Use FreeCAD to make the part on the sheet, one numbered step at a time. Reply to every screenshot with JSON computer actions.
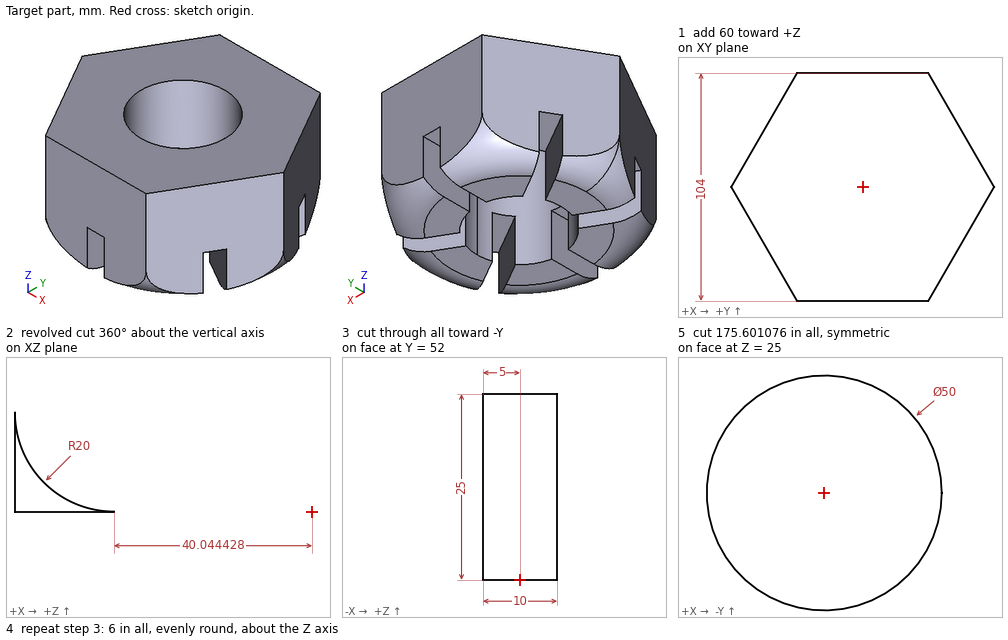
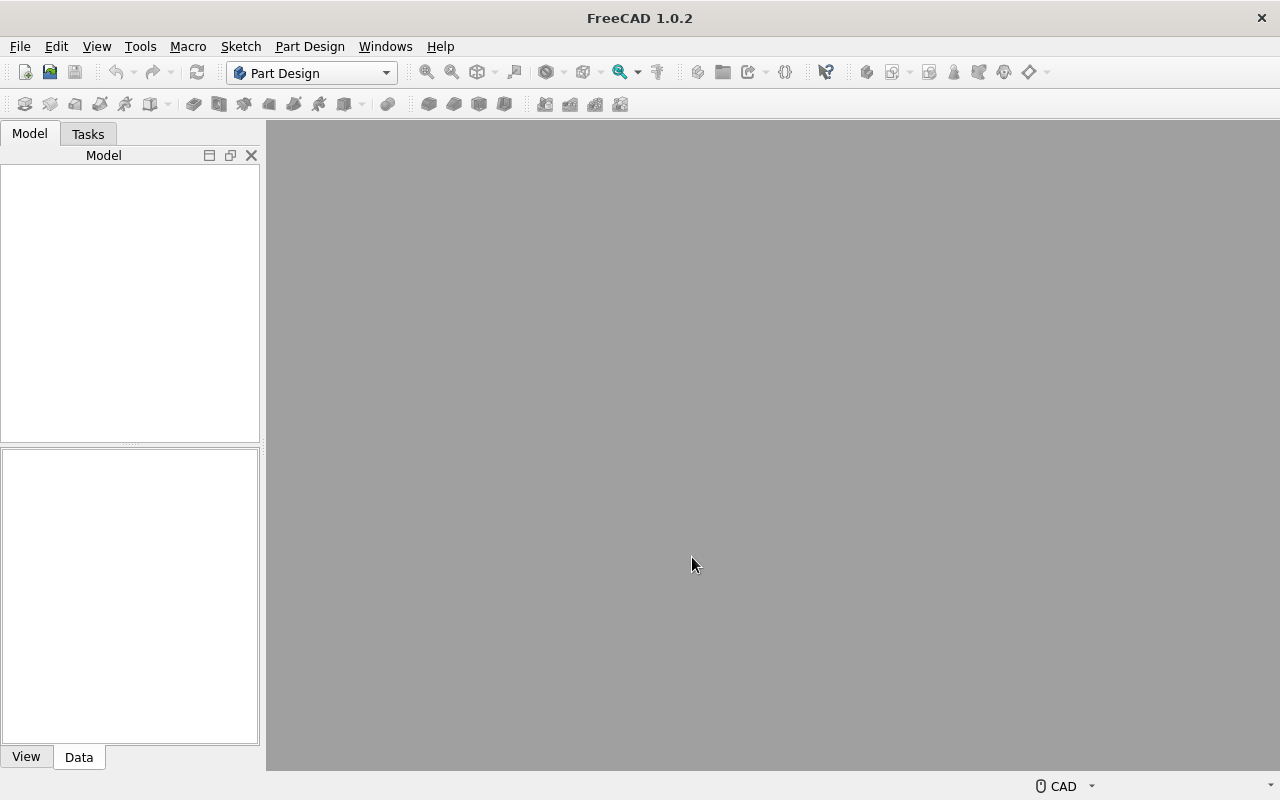
{"action": "left_click", "coordinate": [25, 72]}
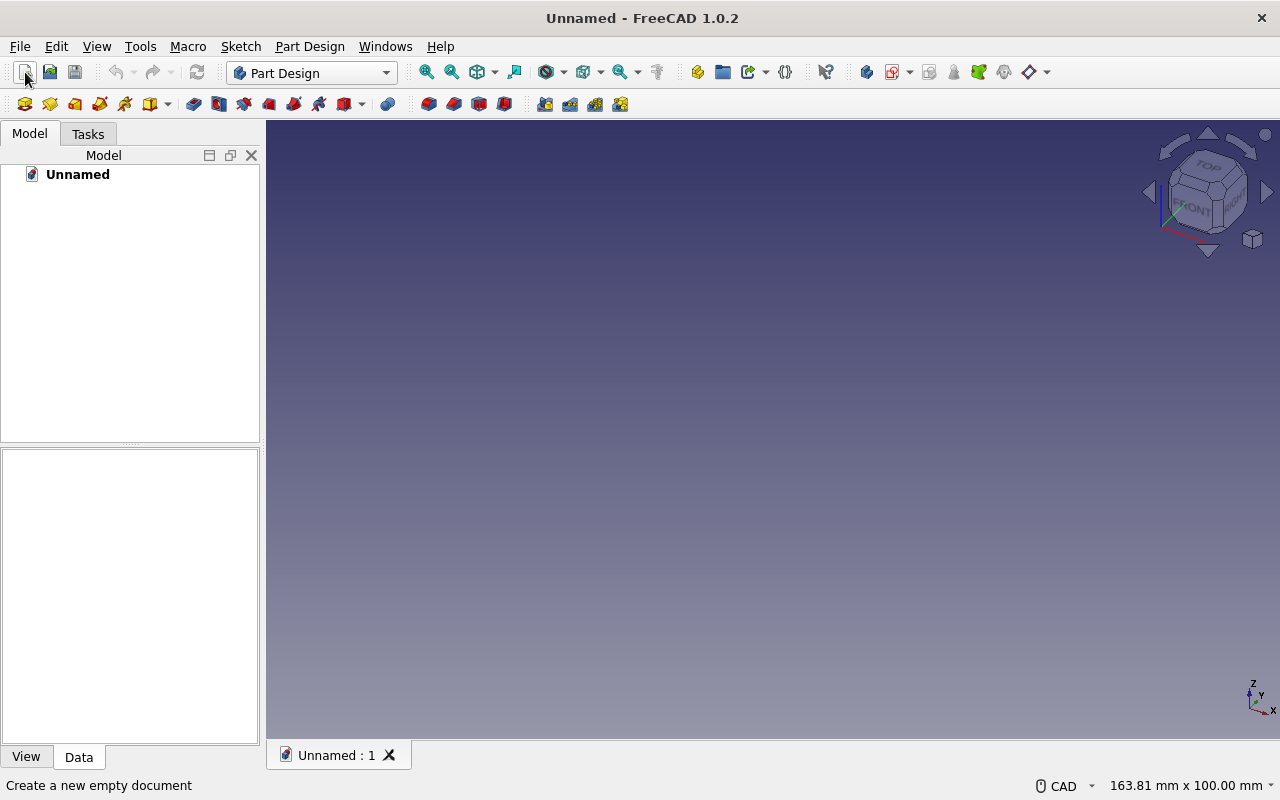
{"action": "left_click", "coordinate": [892, 72]}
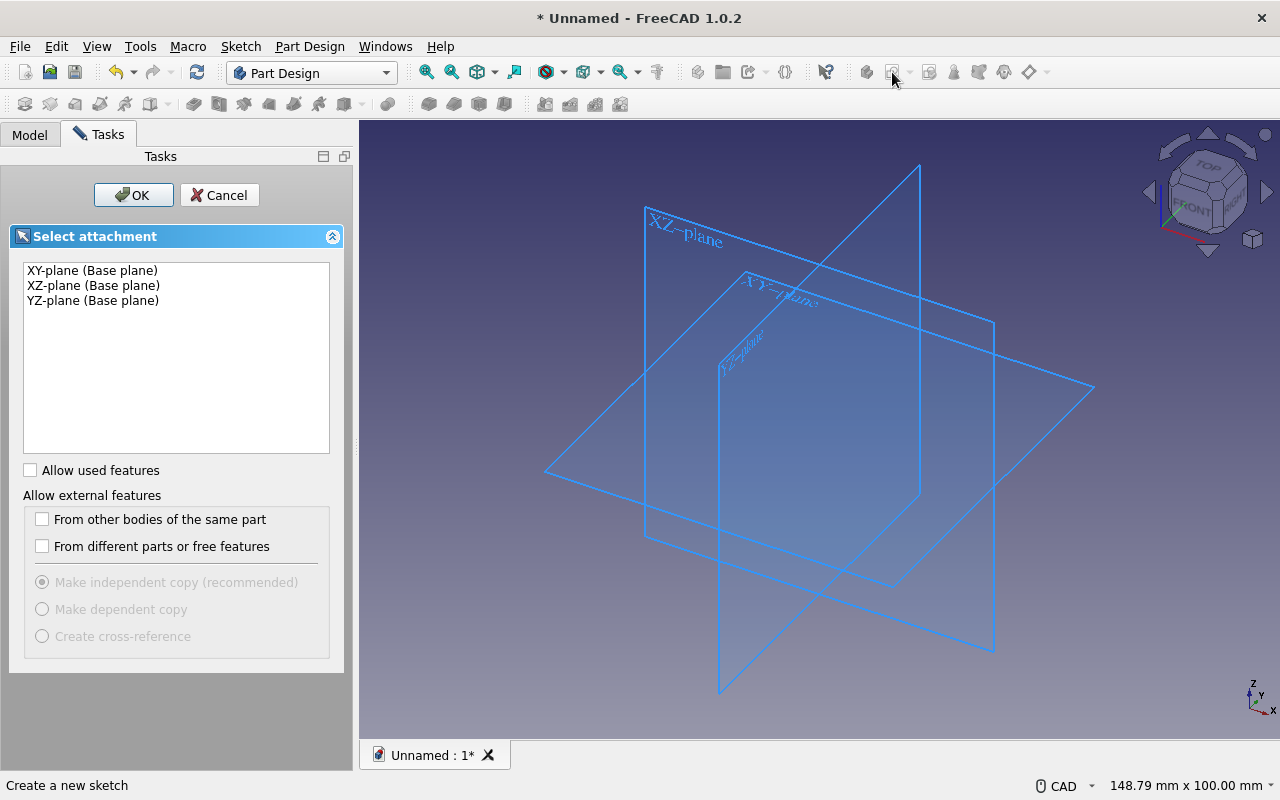
{"action": "left_click", "coordinate": [84, 270]}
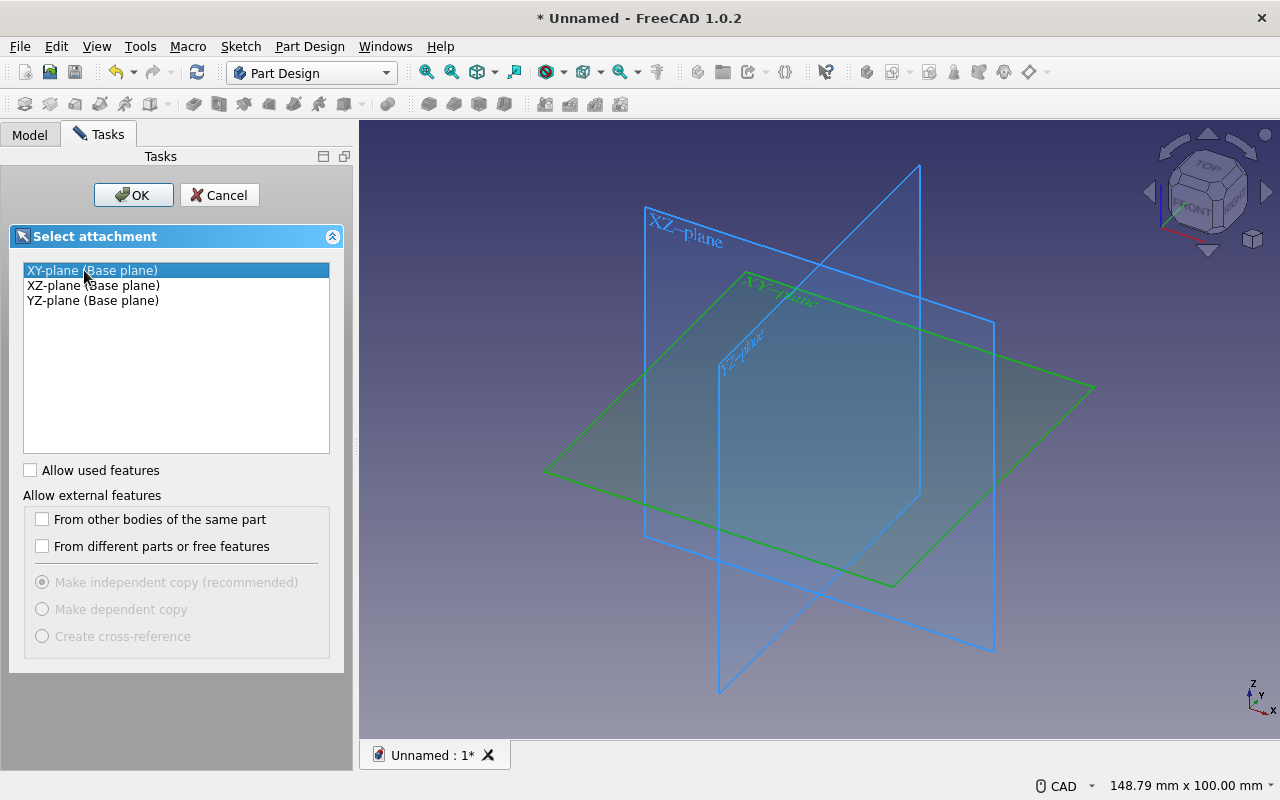
{"action": "left_click", "coordinate": [134, 195]}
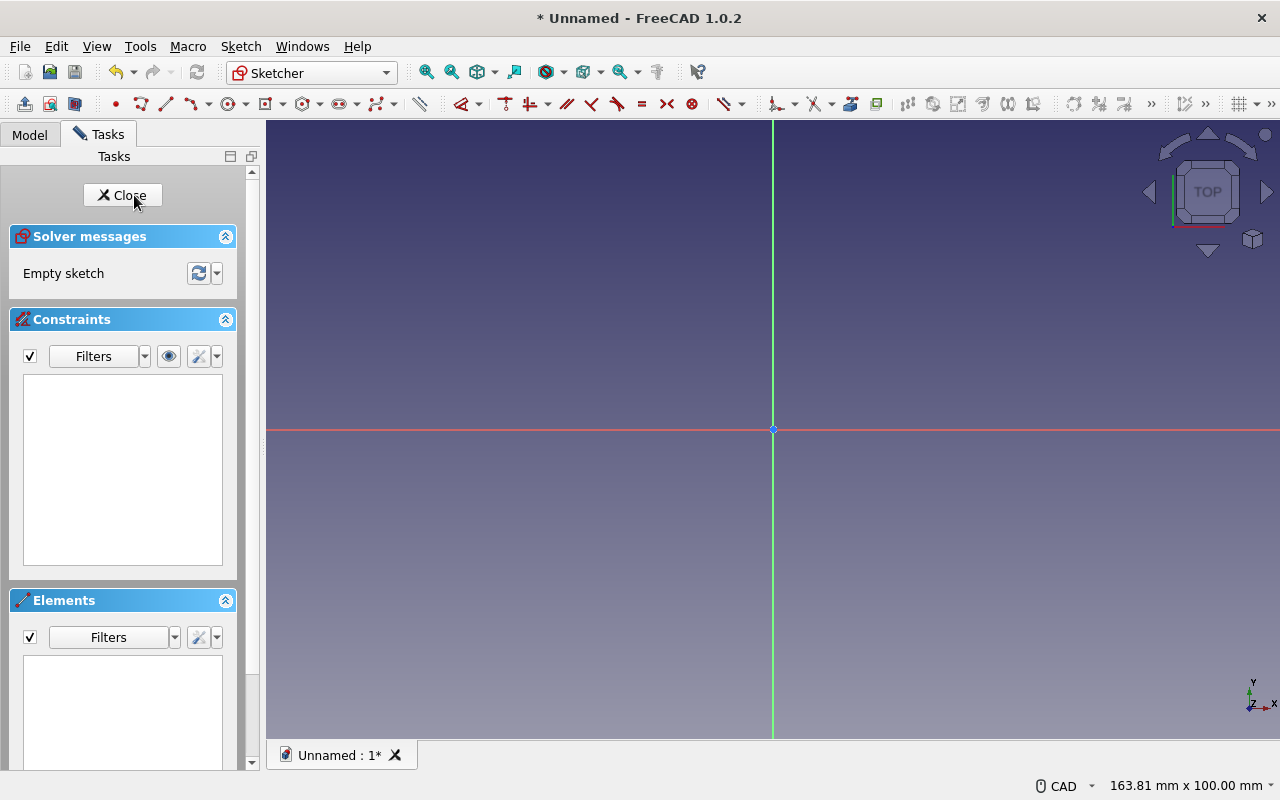
{"action": "scroll", "coordinate": [565, 429], "scroll_direction": "down", "scroll_amount": 2}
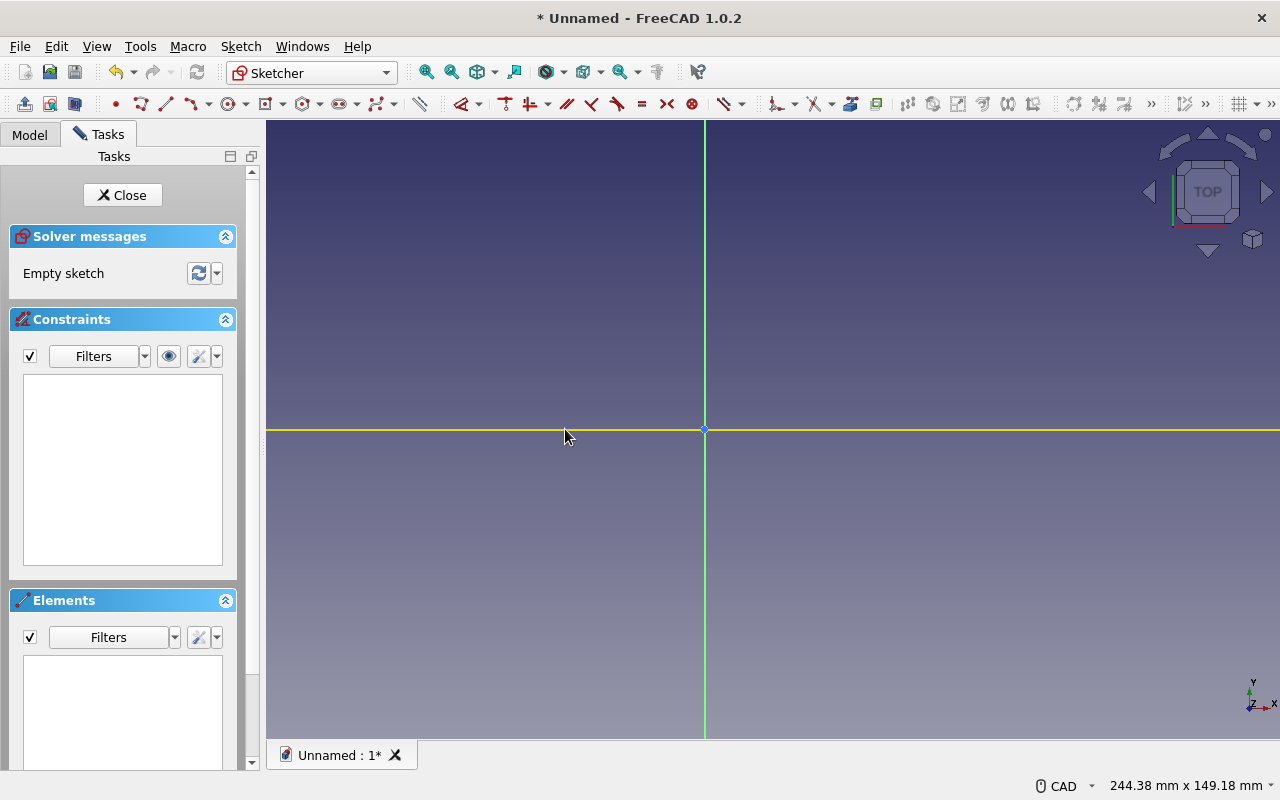
{"action": "left_click", "coordinate": [302, 104]}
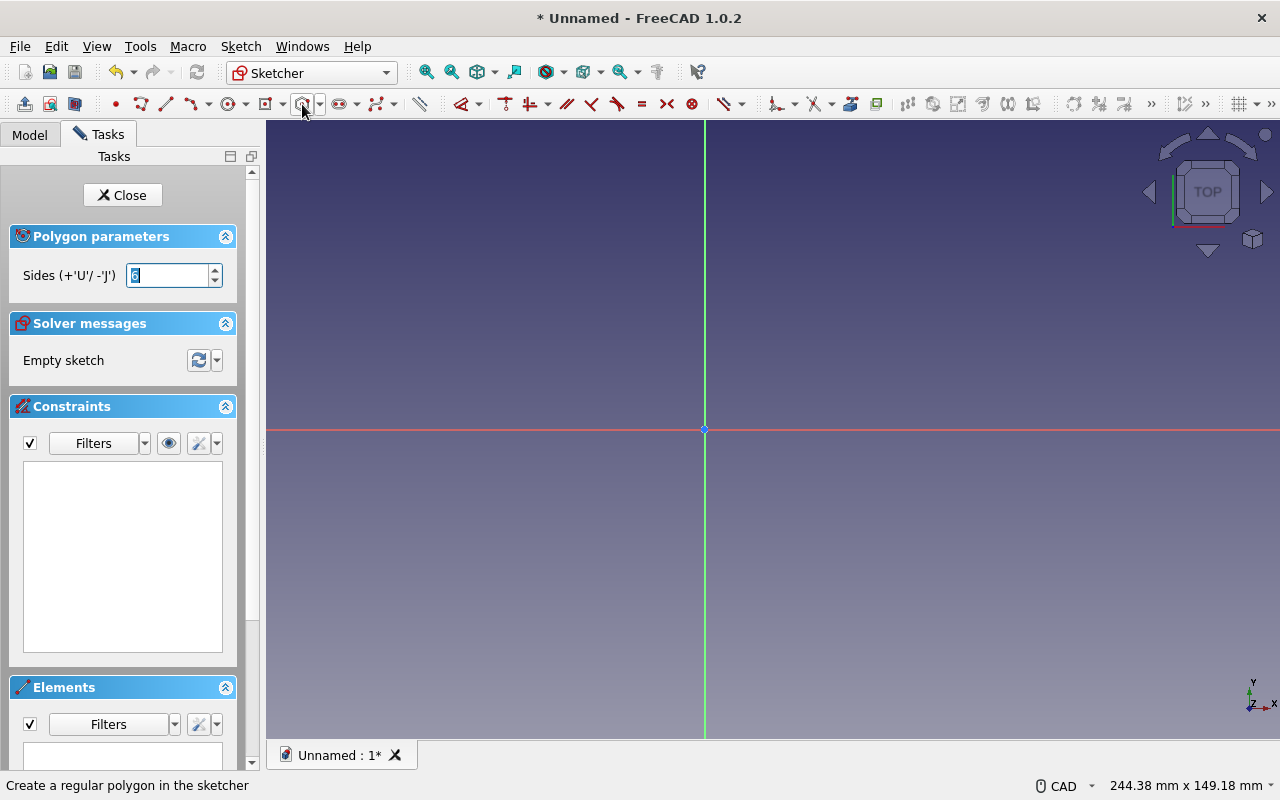
{"action": "left_click", "coordinate": [705, 430]}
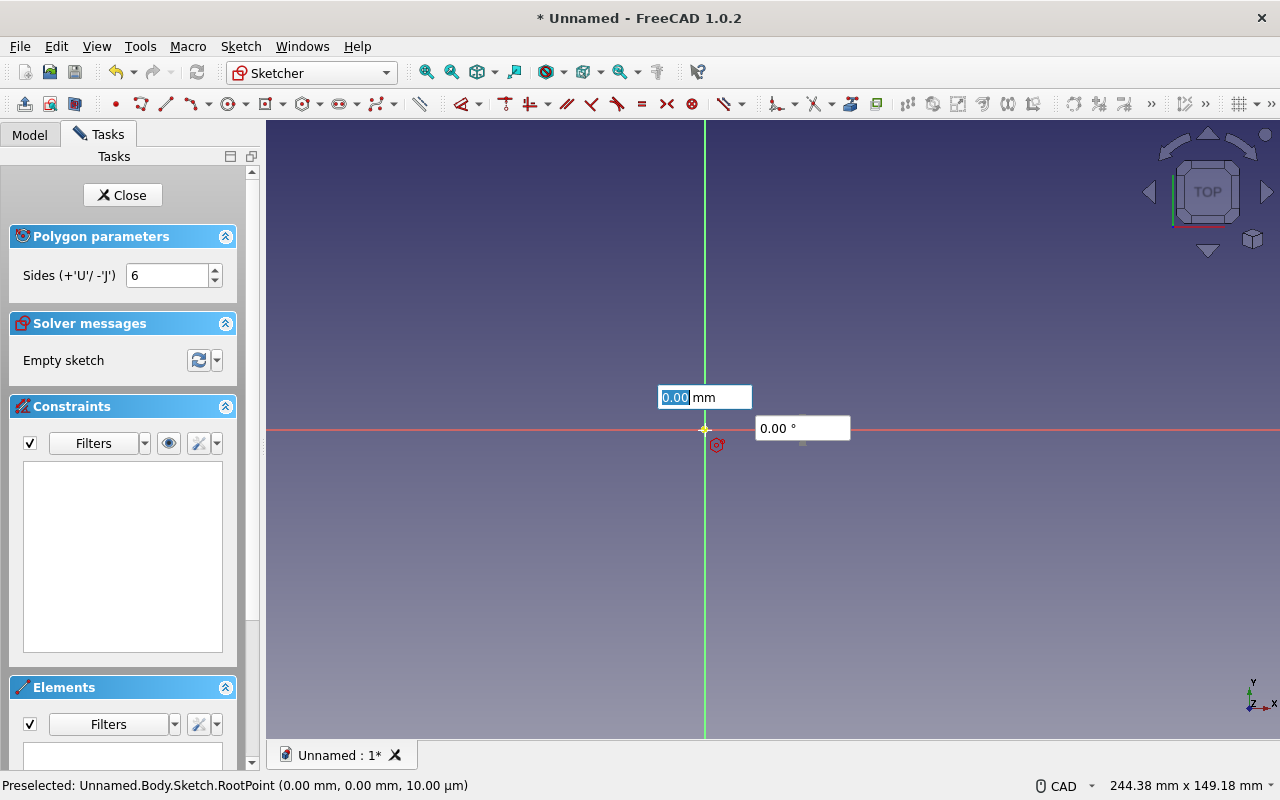
{"action": "left_click", "coordinate": [954, 430]}
{"action": "key", "text": "Escape"}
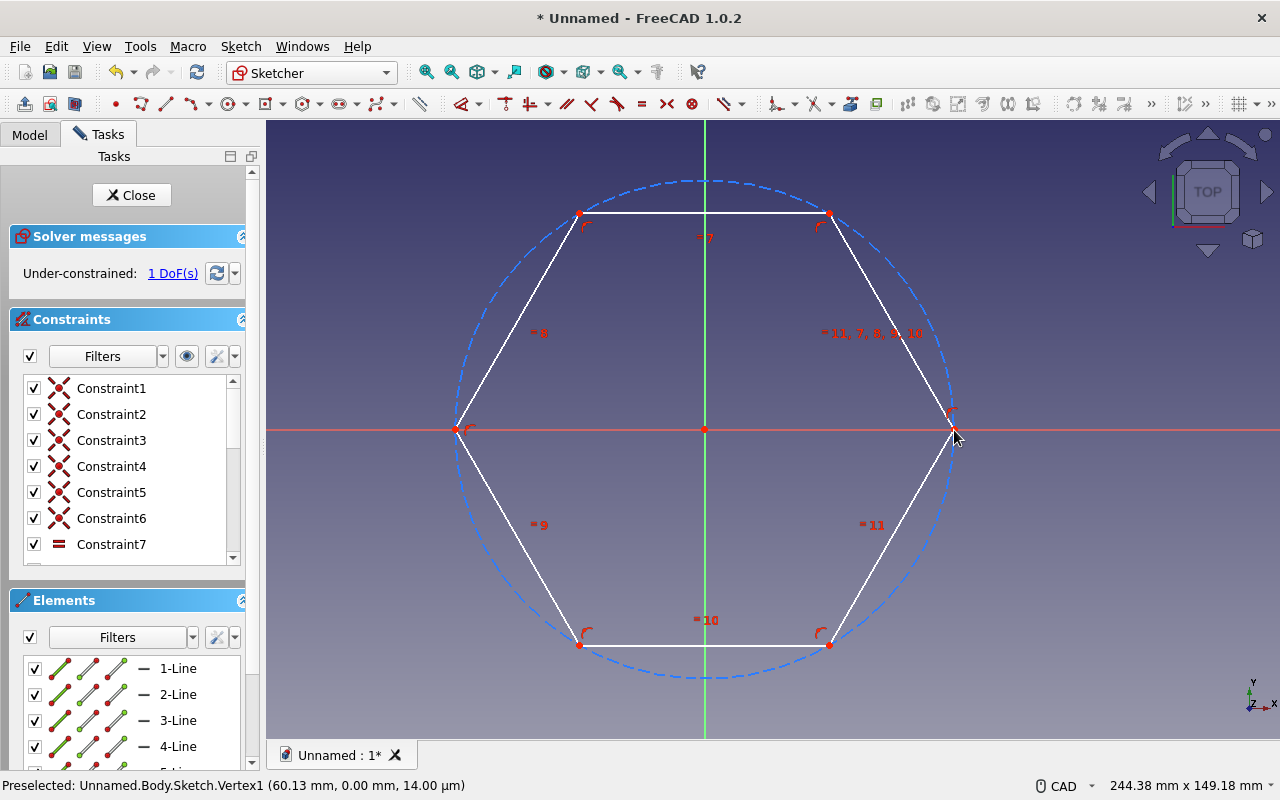
{"action": "key", "text": "d"}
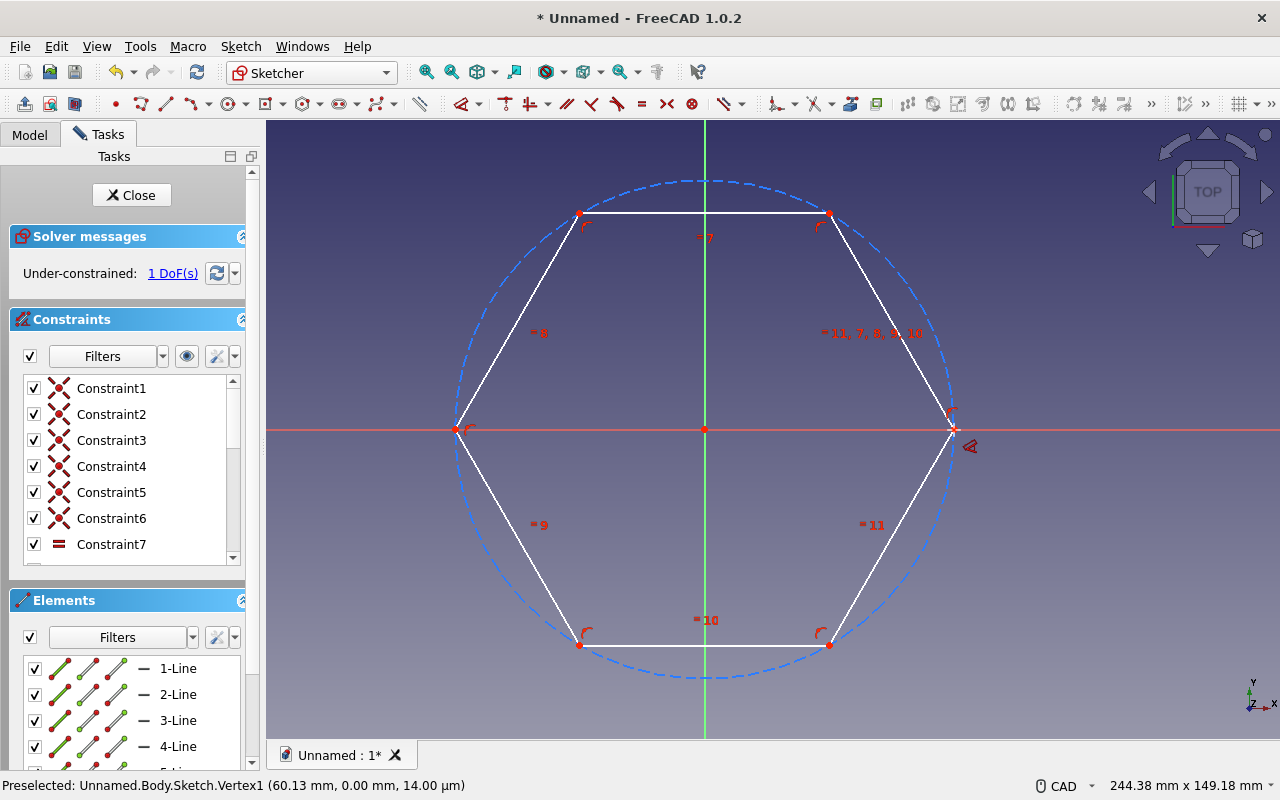
{"action": "left_click", "coordinate": [580, 646]}